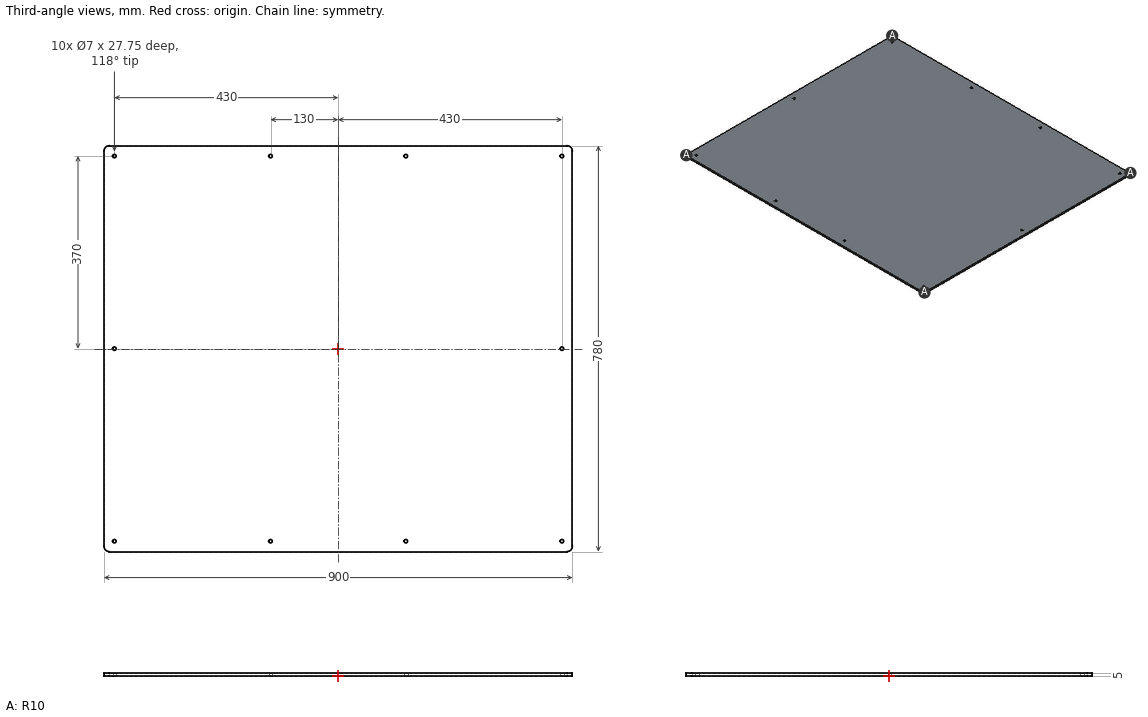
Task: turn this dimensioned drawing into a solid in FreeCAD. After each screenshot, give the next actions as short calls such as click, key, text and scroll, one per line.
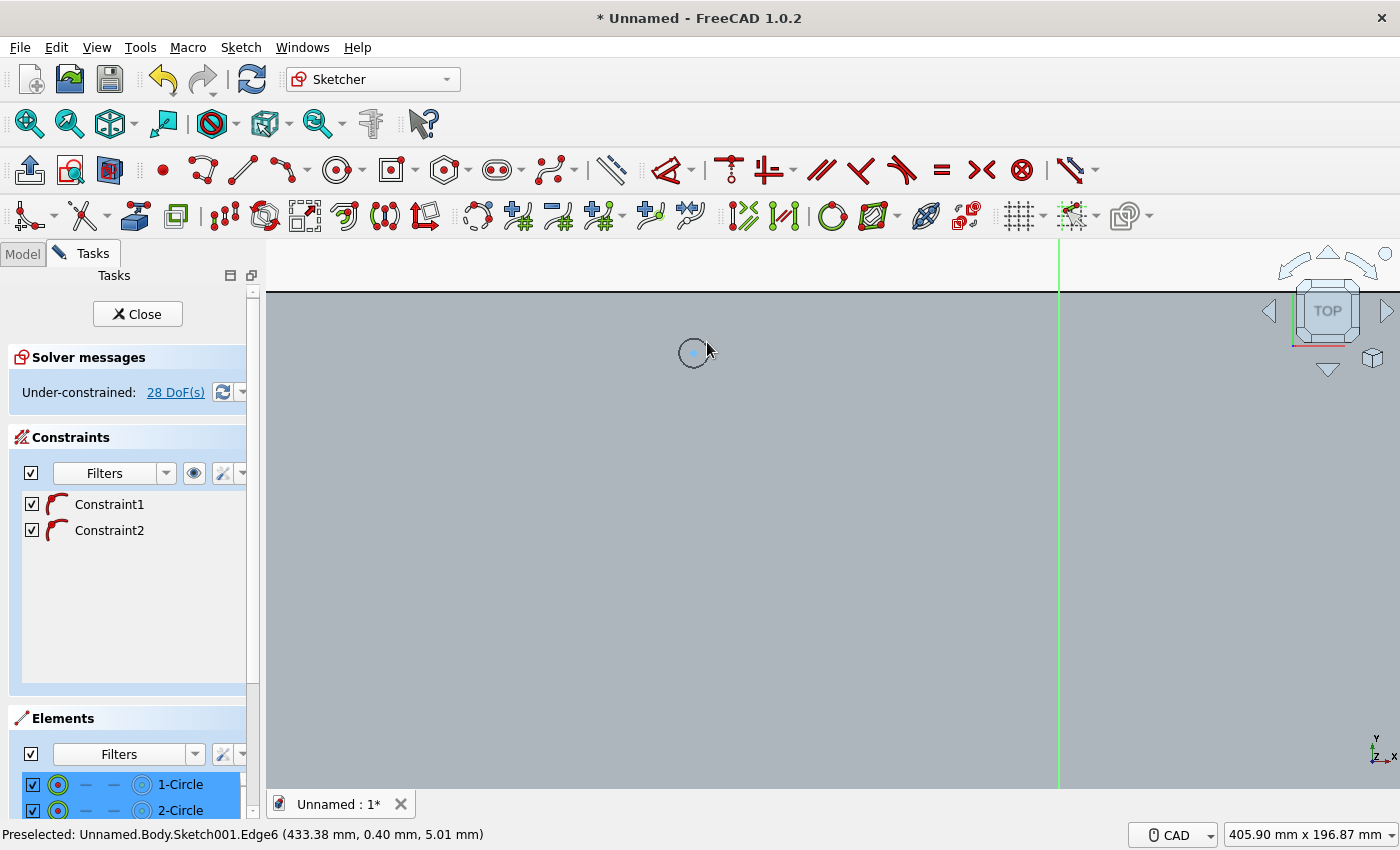
click(704, 343)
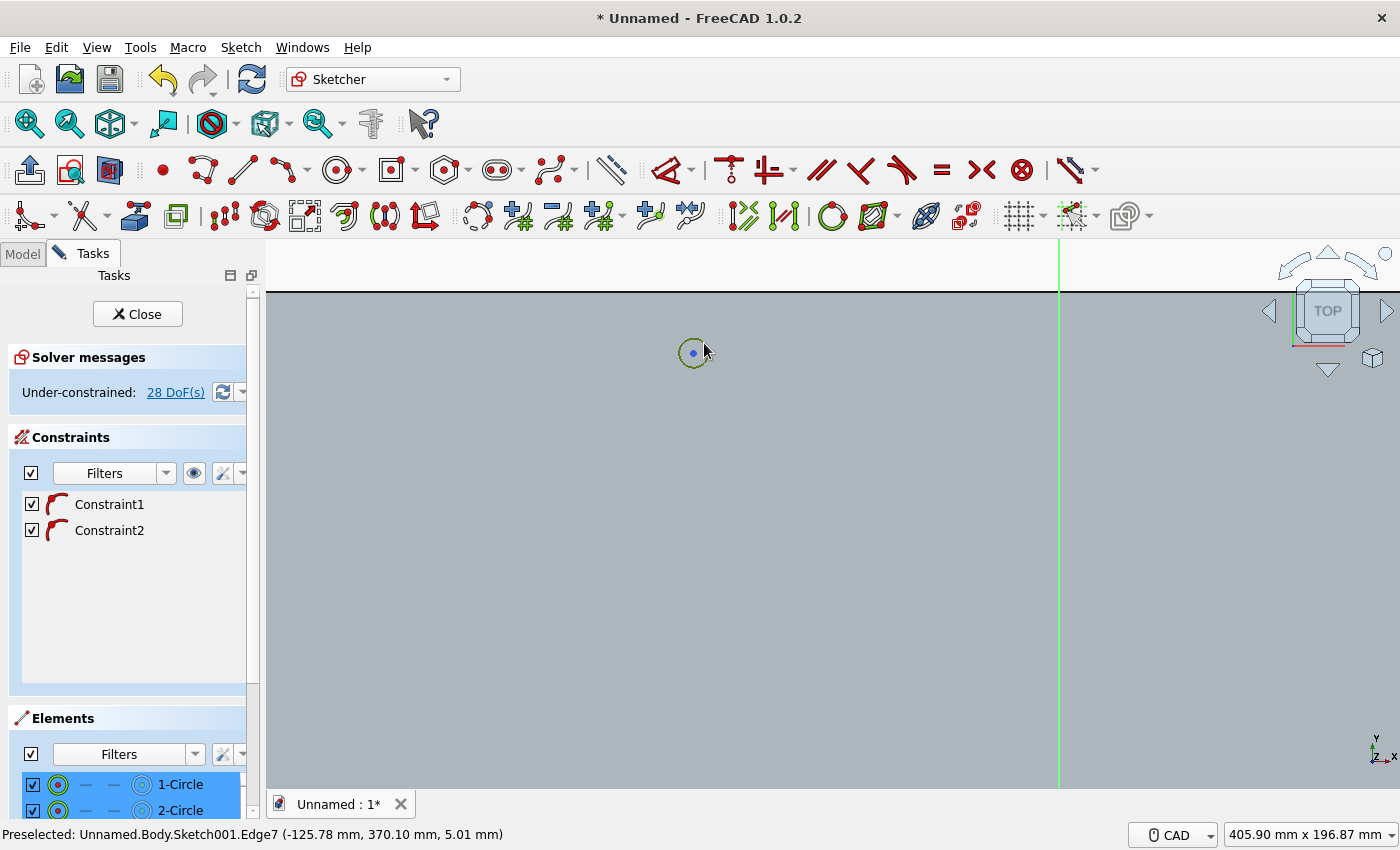
scroll(706, 342, down, 9)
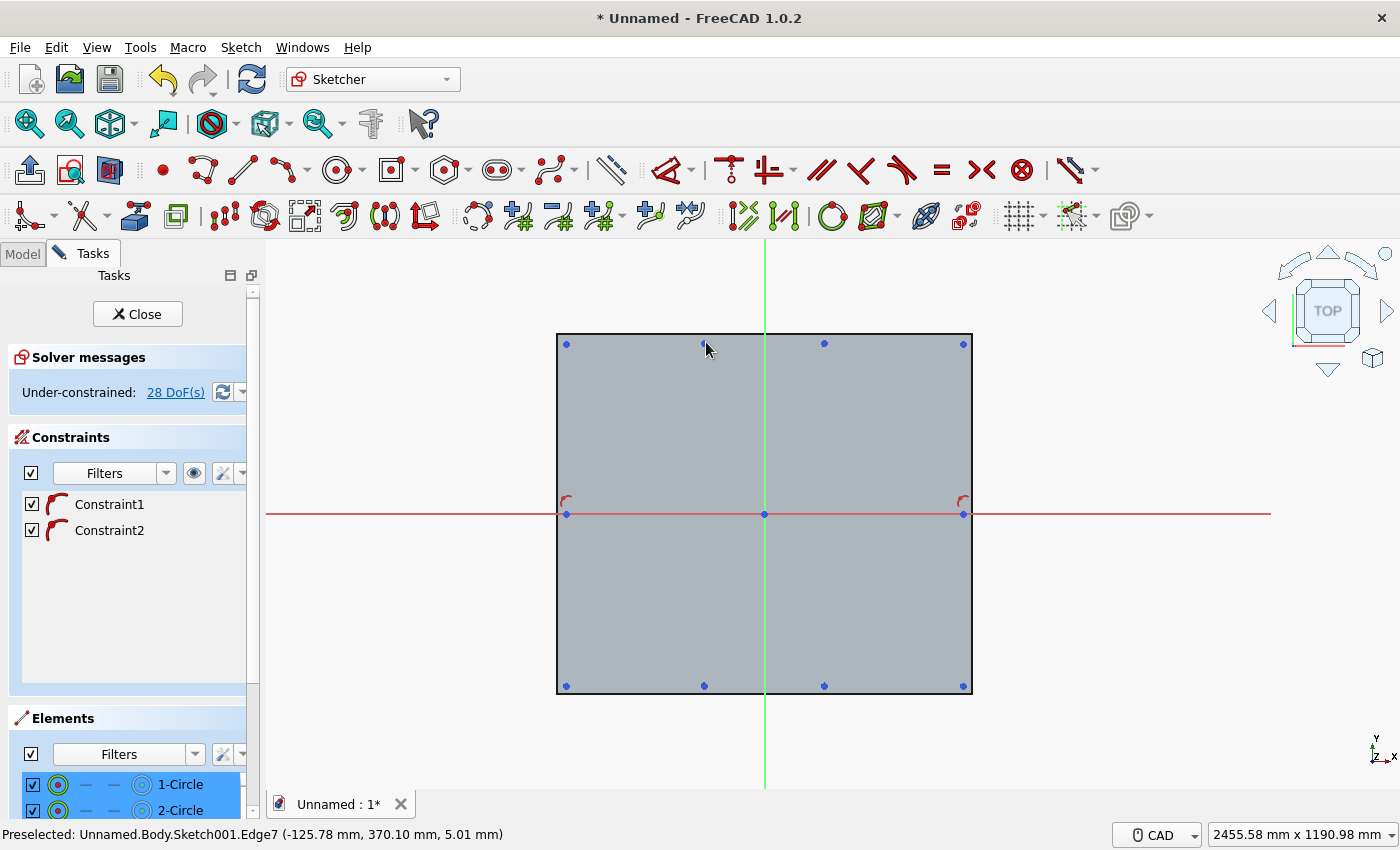
scroll(826, 342, up, 9)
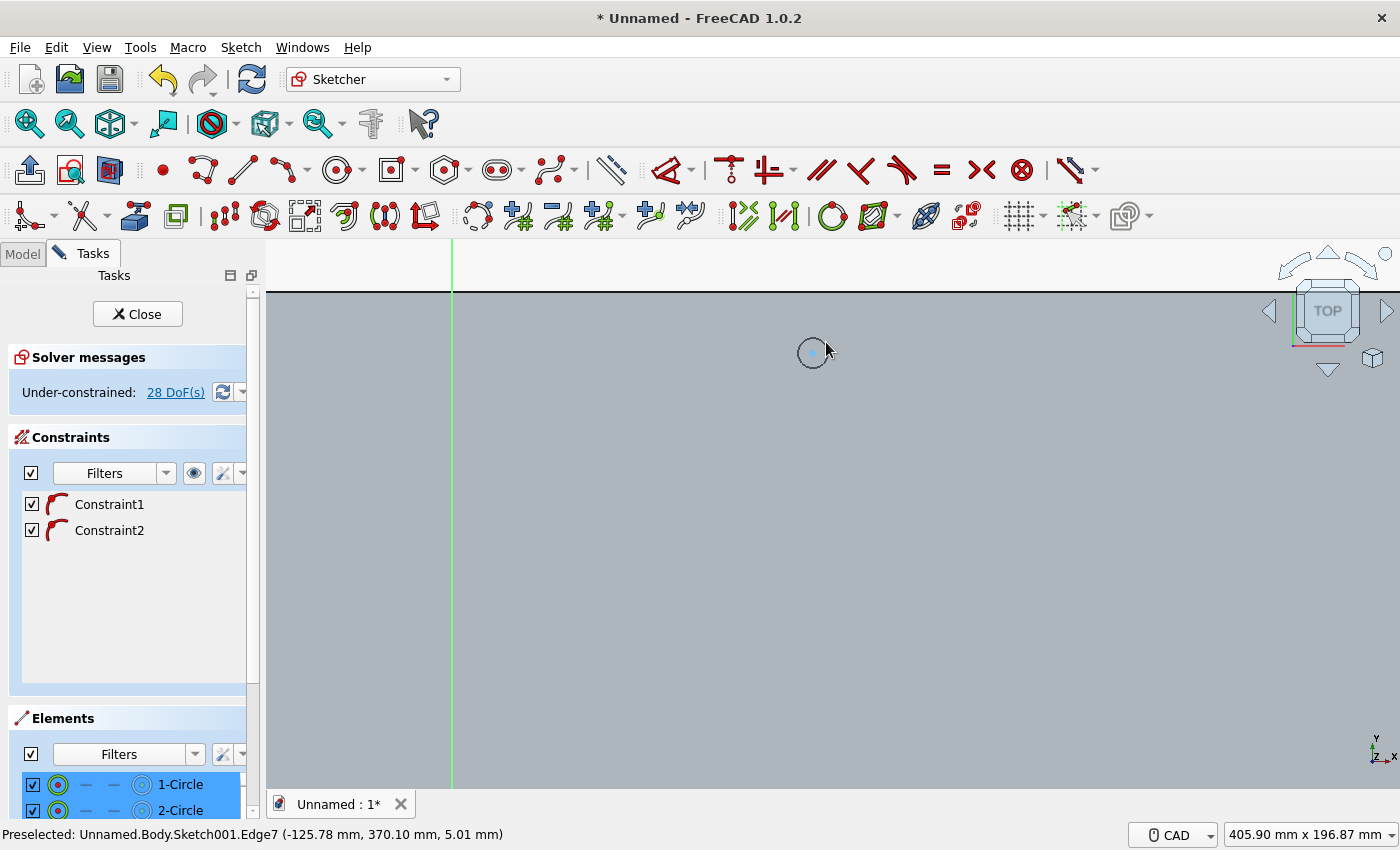
click(823, 343)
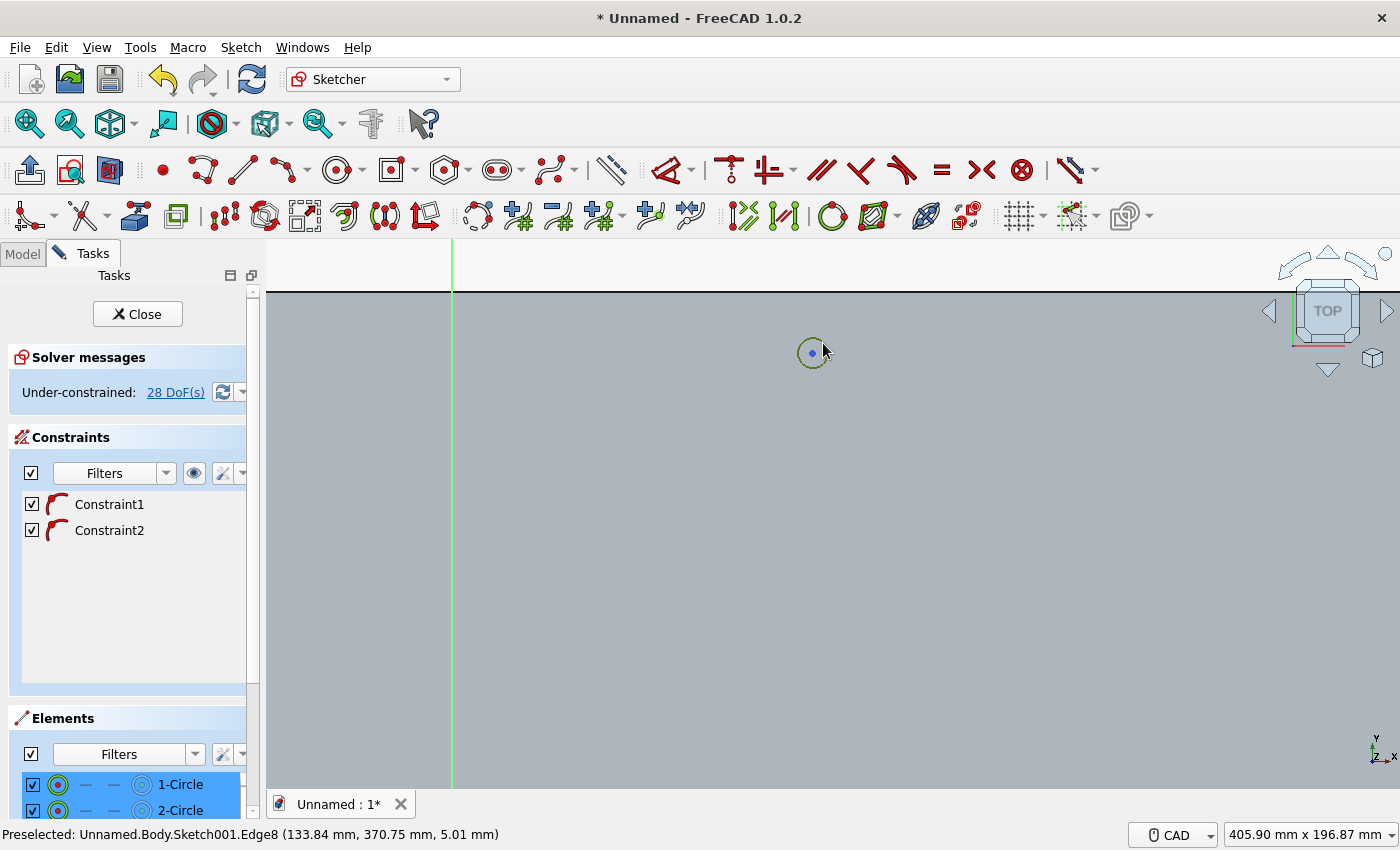
scroll(826, 342, down, 9)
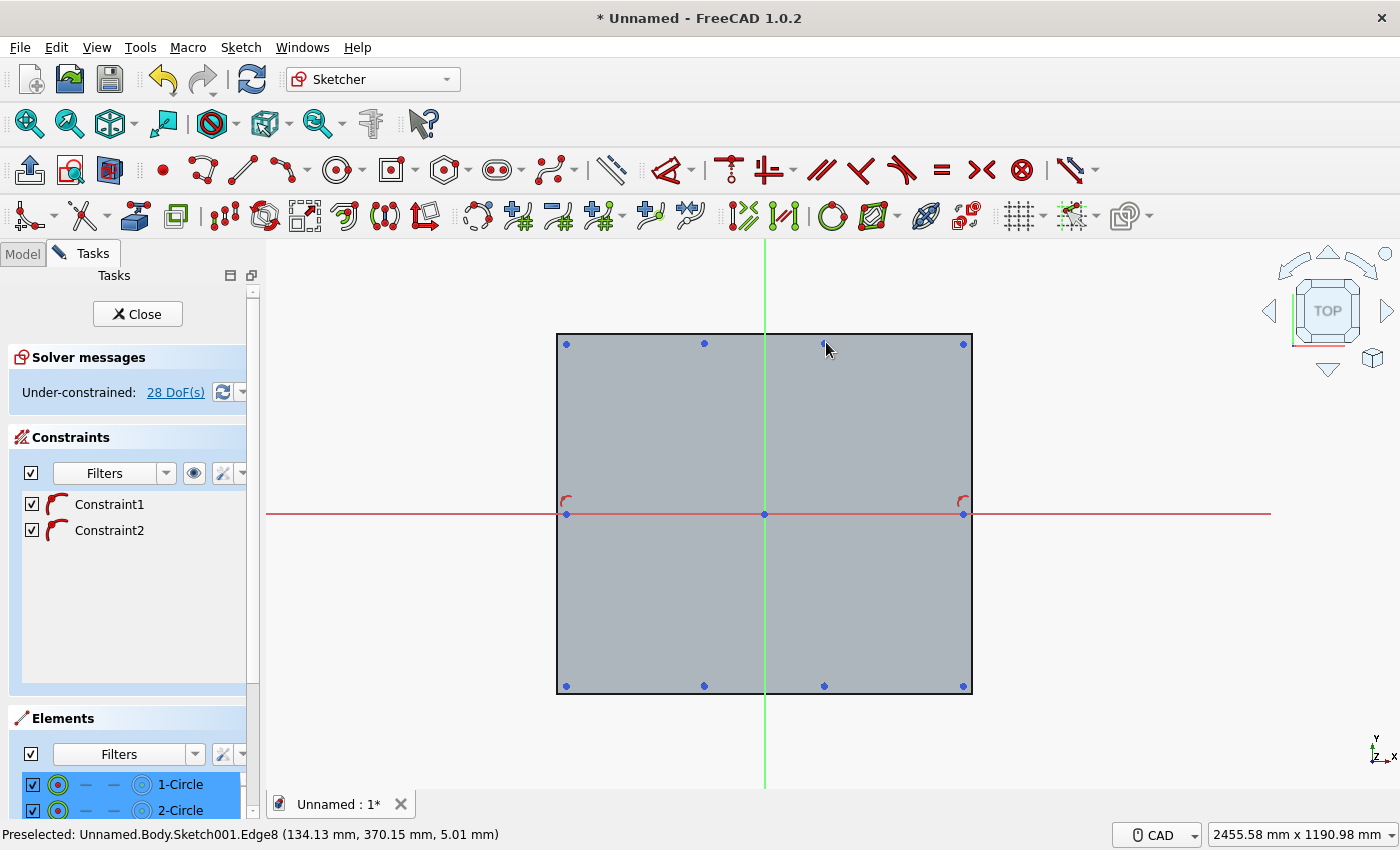
scroll(706, 684, up, 9)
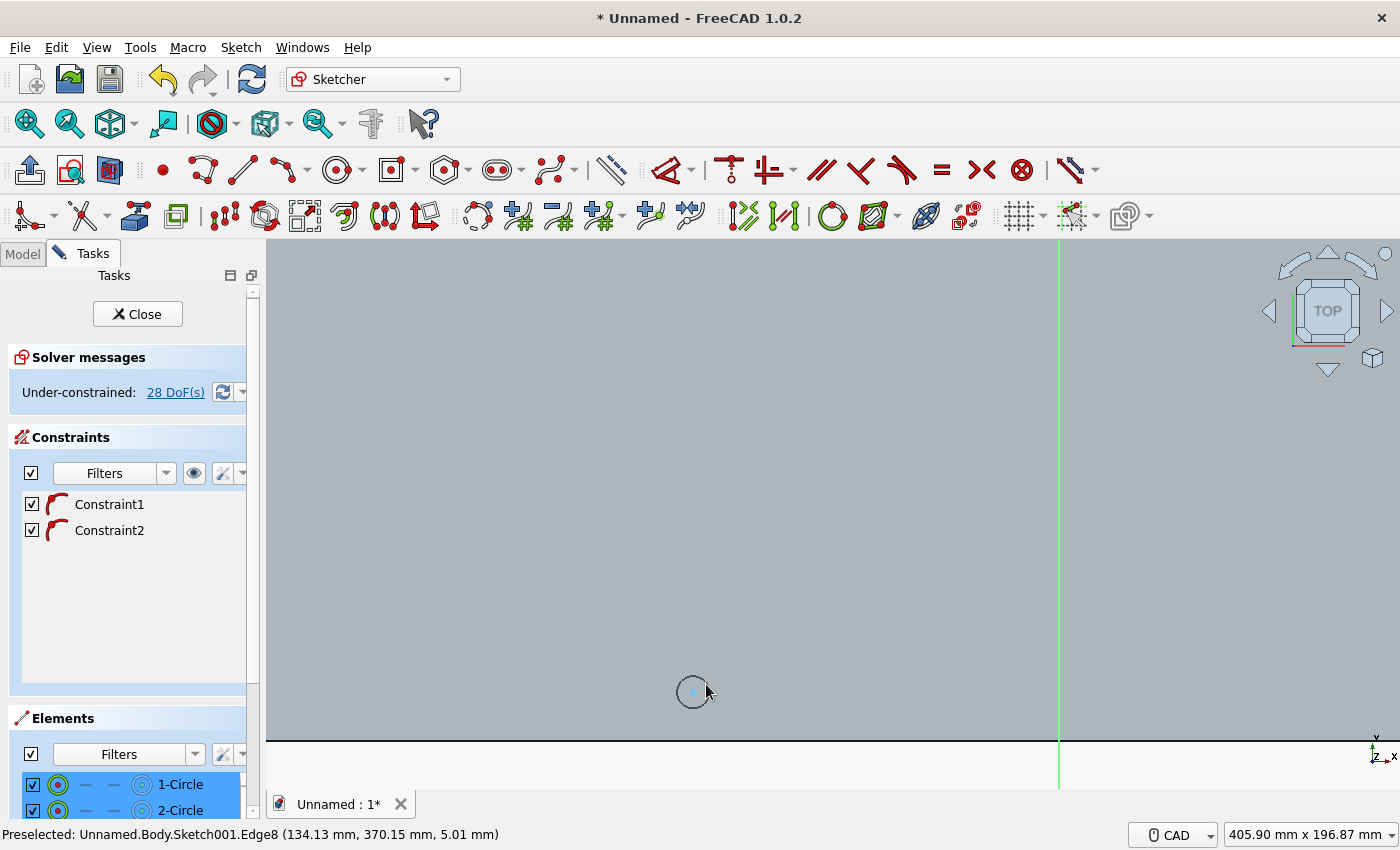
click(704, 681)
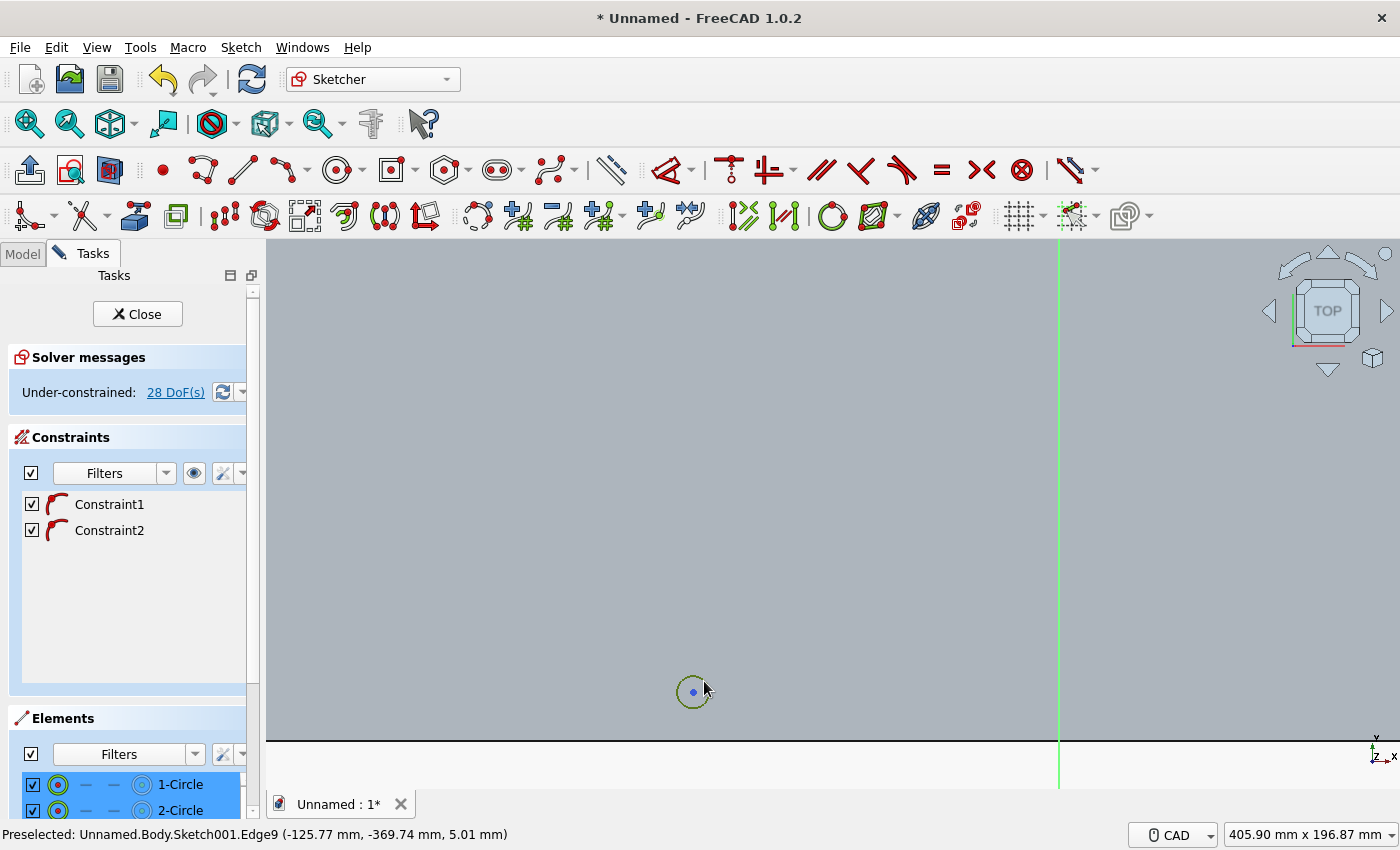
scroll(706, 685, down, 9)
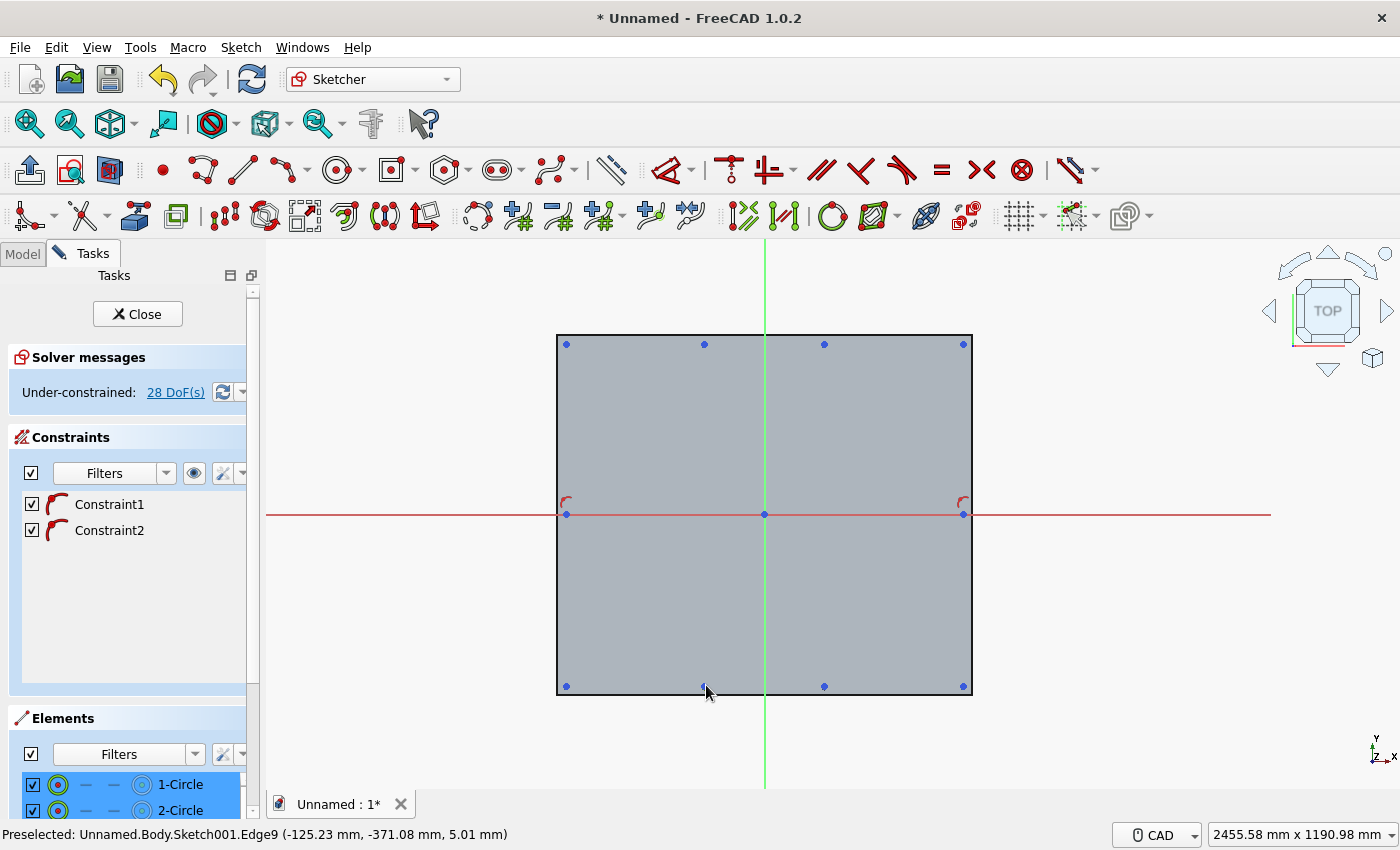
scroll(826, 685, up, 9)